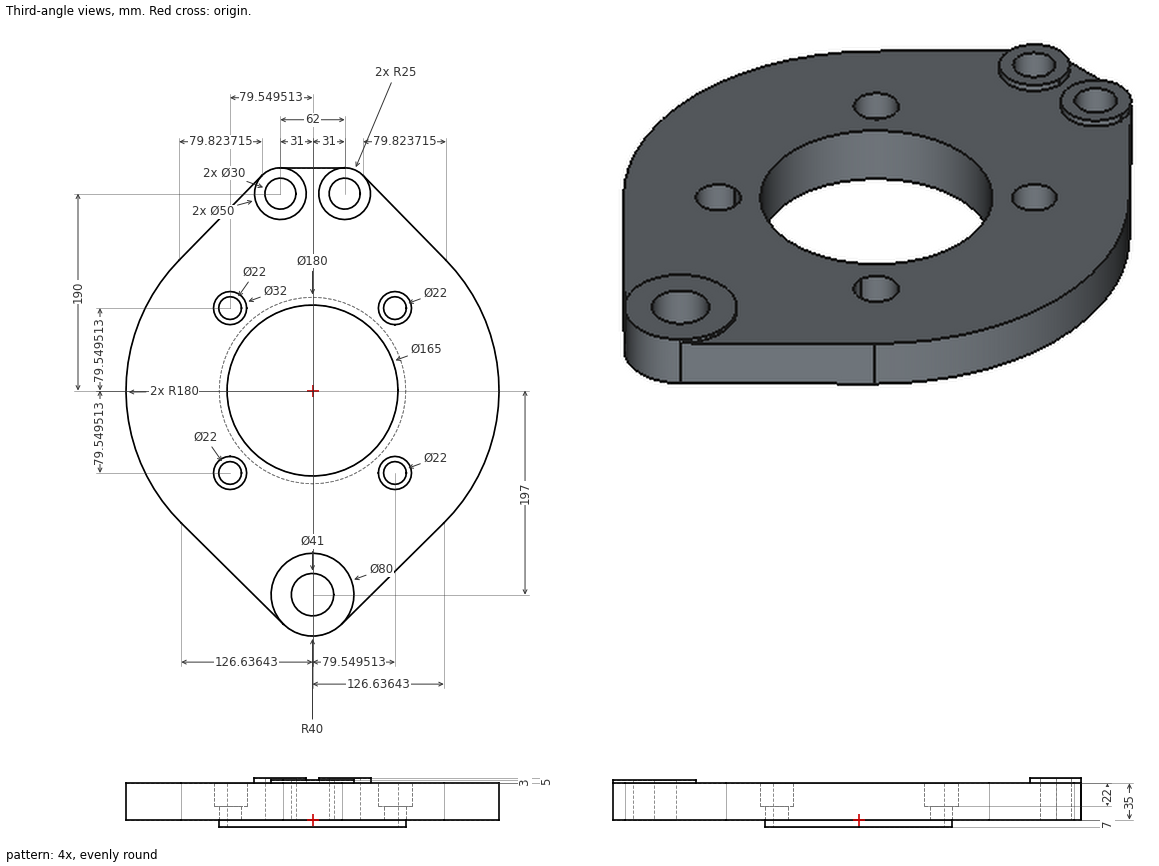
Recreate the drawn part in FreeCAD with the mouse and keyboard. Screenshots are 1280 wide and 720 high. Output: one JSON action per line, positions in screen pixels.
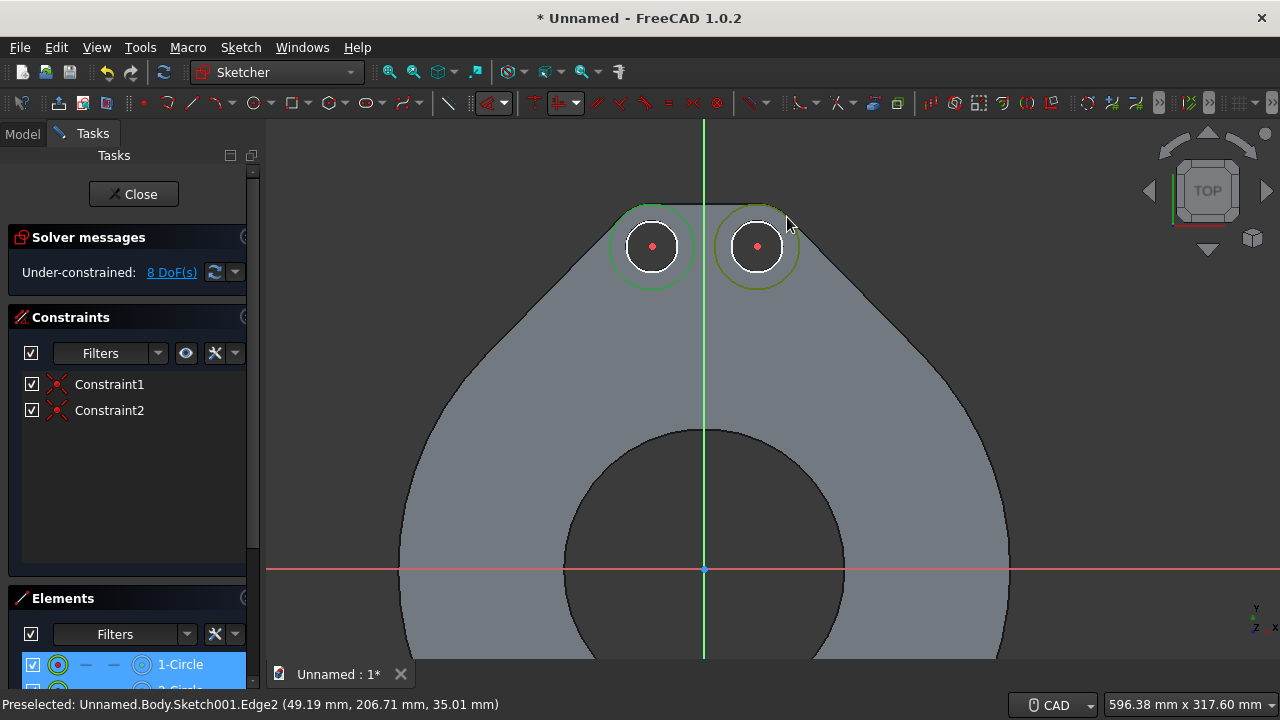
{"action": "left_click", "coordinate": [670, 104]}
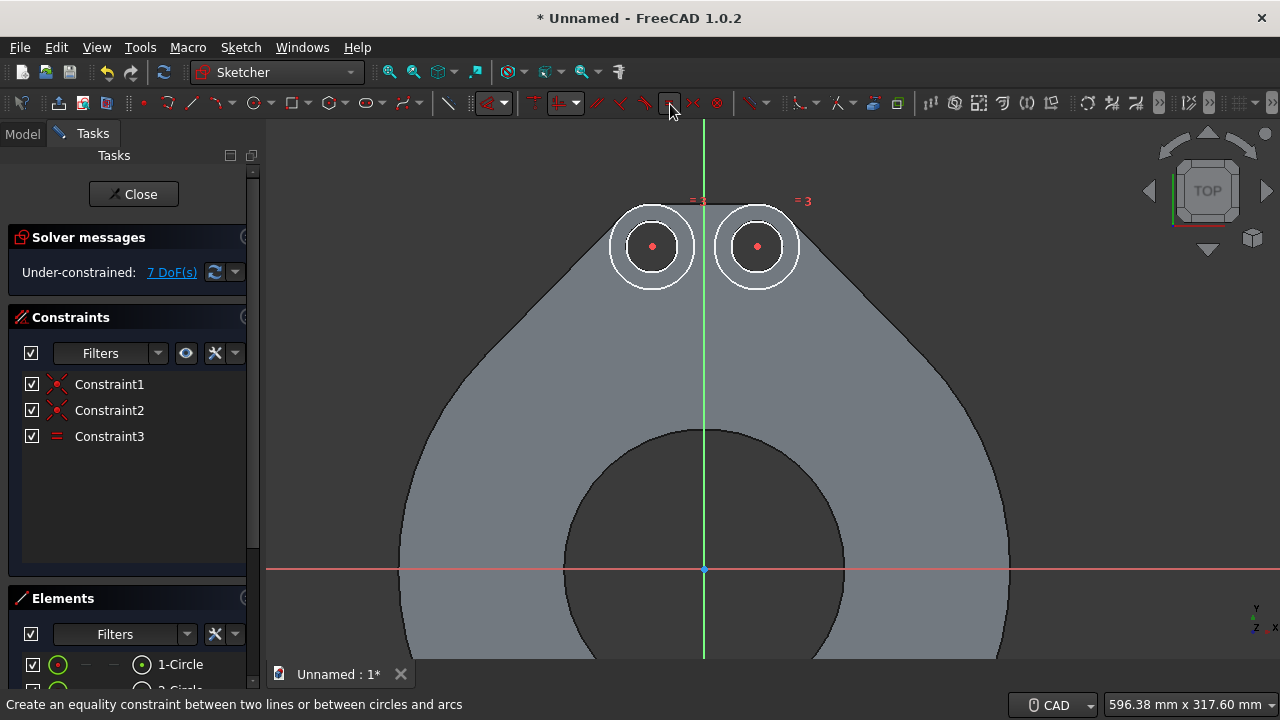
{"action": "left_click", "coordinate": [670, 229]}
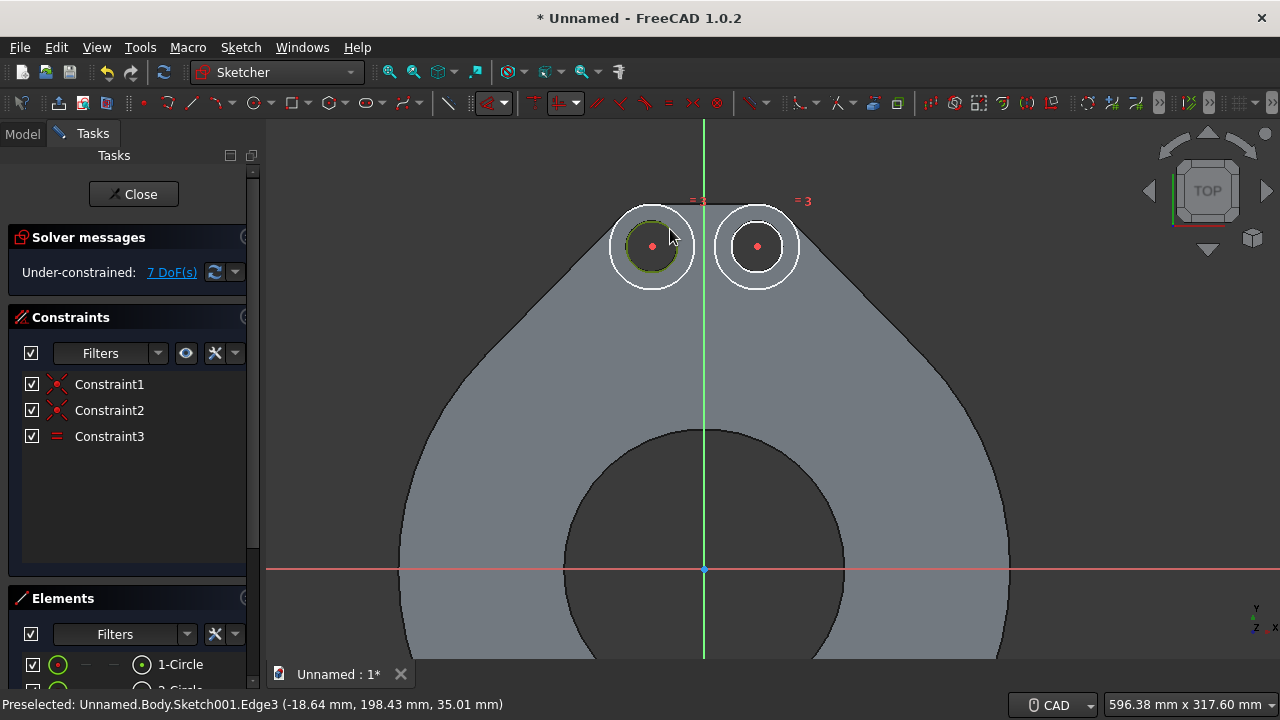
{"action": "left_click", "coordinate": [775, 229]}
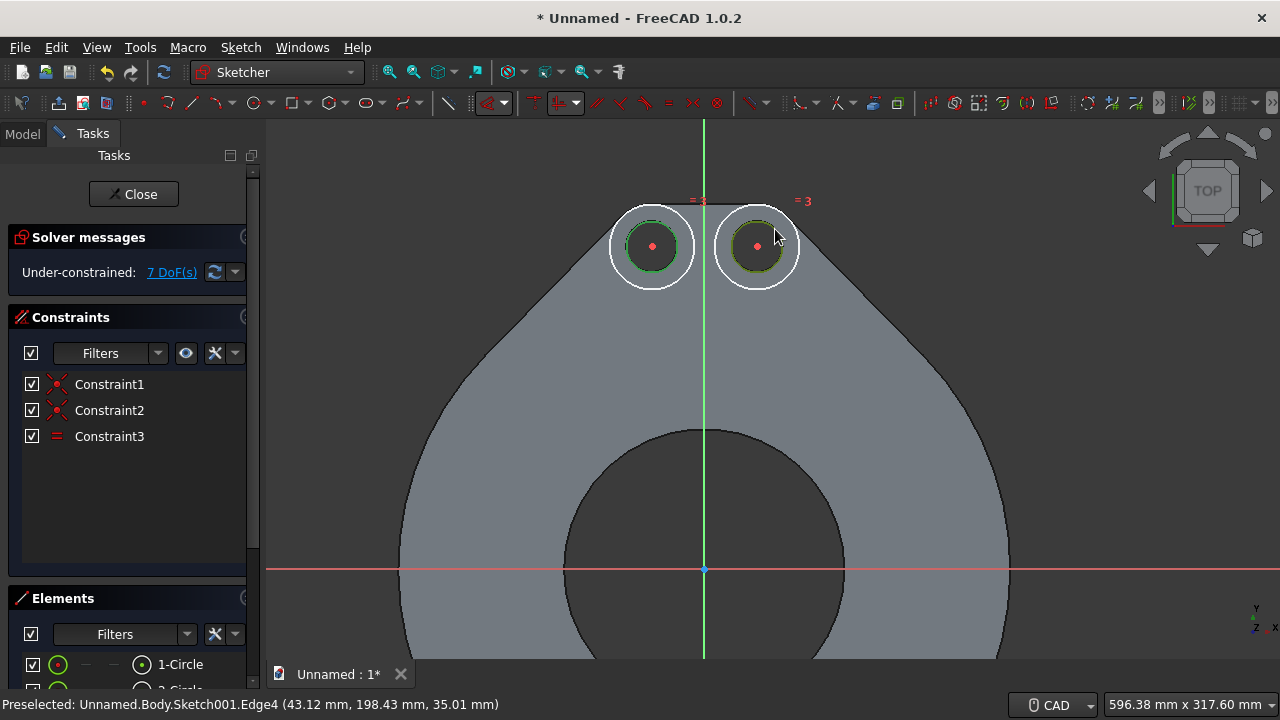
{"action": "key", "text": "e"}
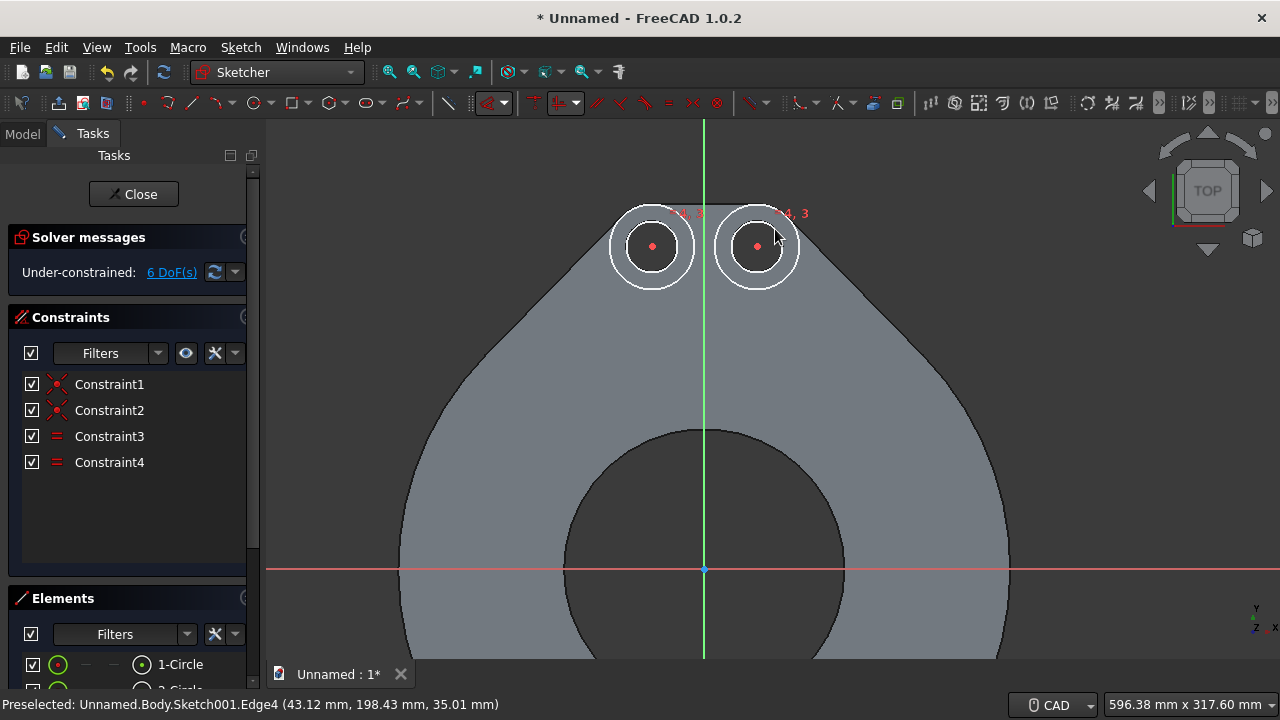
{"action": "left_click", "coordinate": [652, 247]}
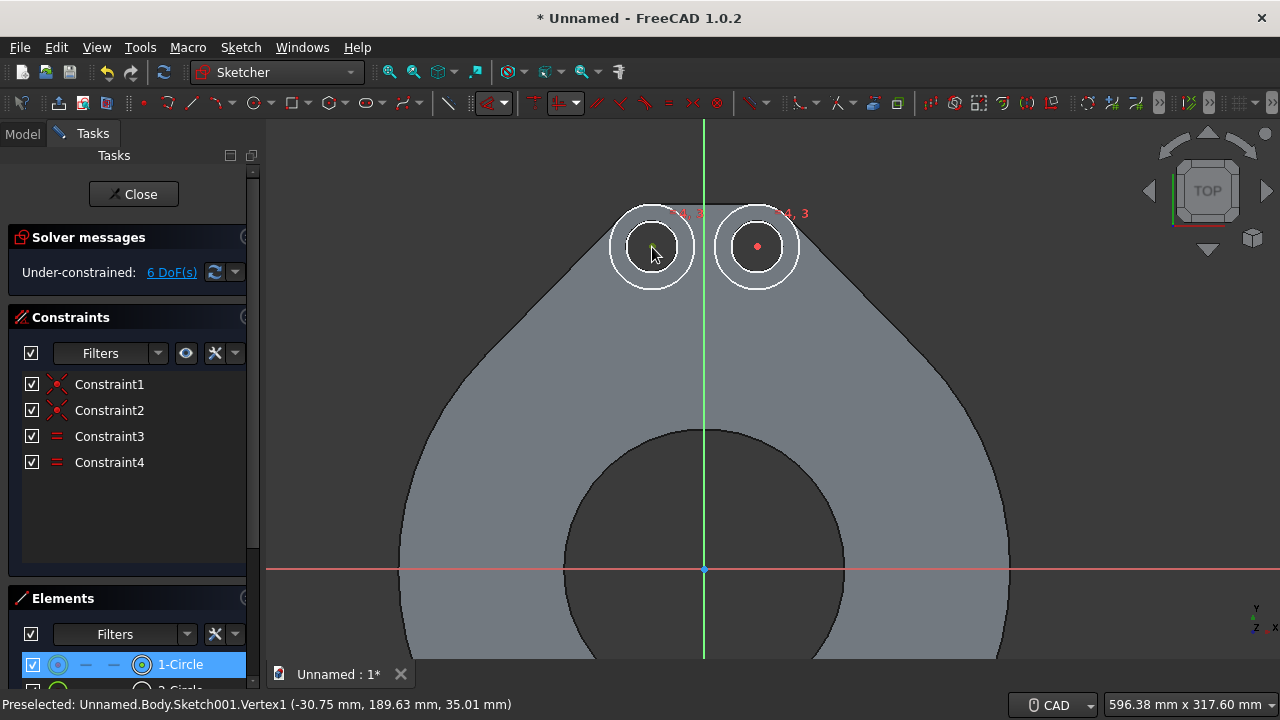
{"action": "left_click", "coordinate": [757, 247]}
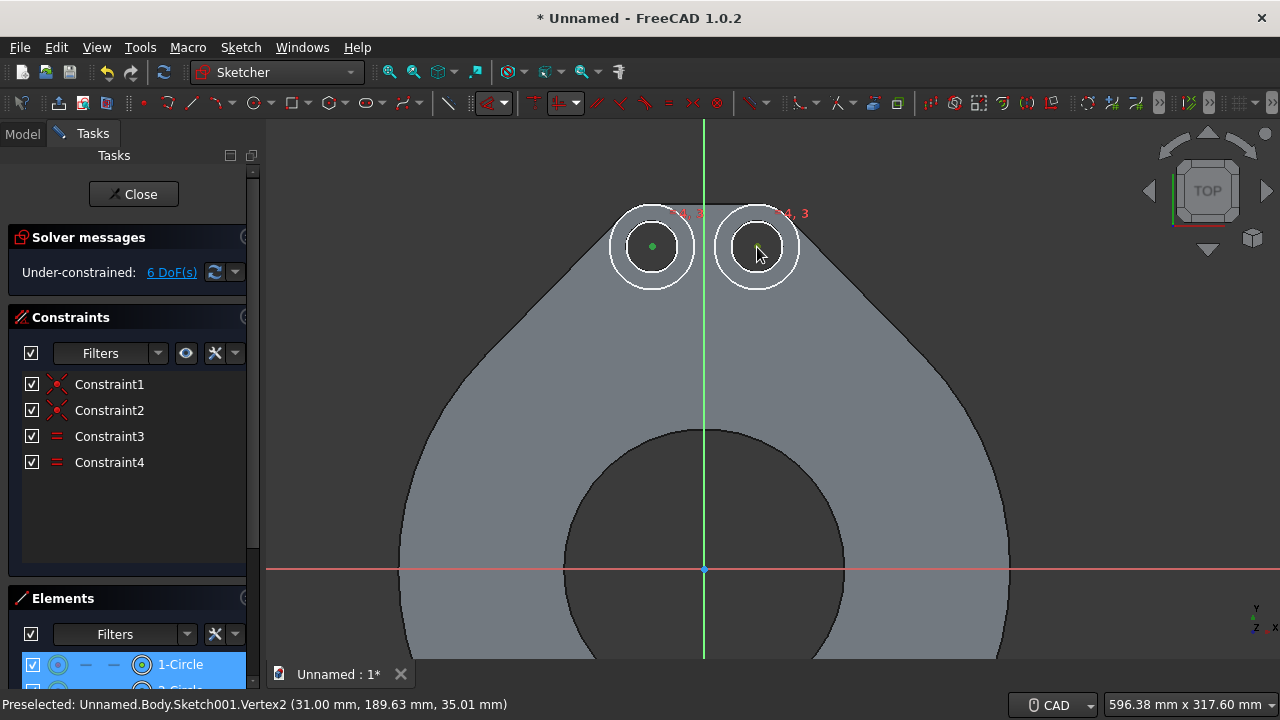
{"action": "key", "text": "h"}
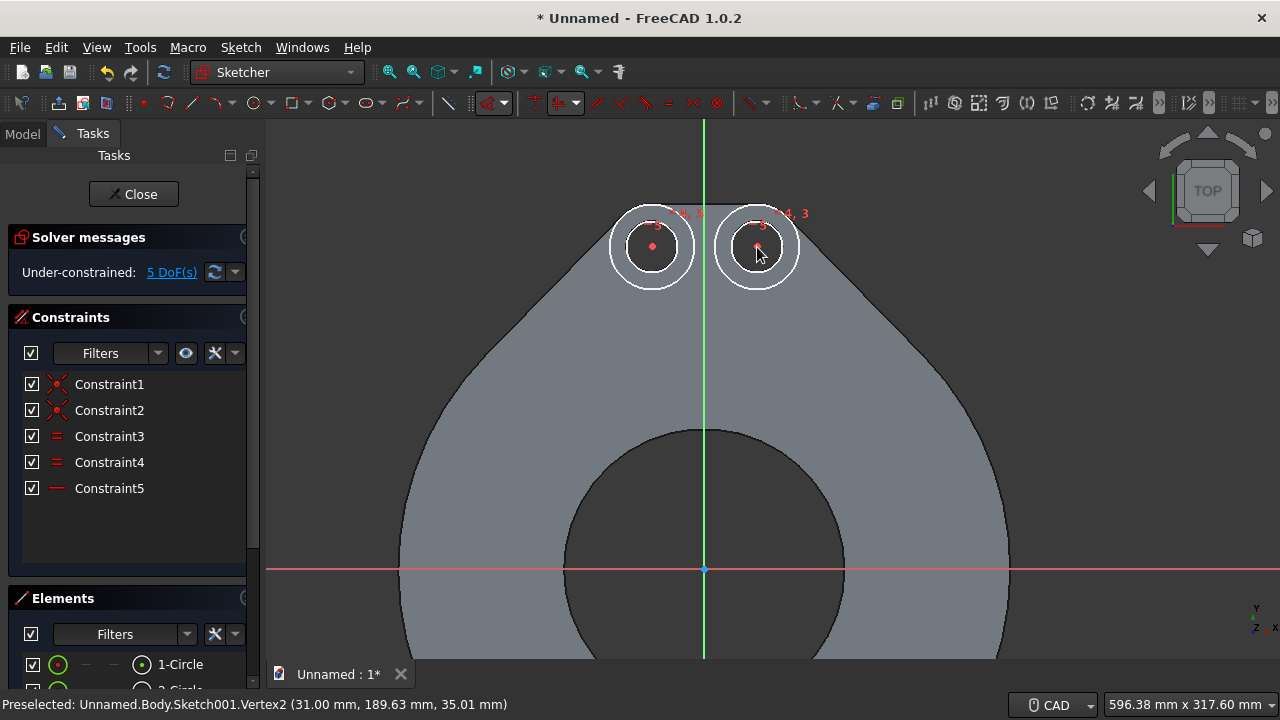
{"action": "left_click", "coordinate": [622, 217]}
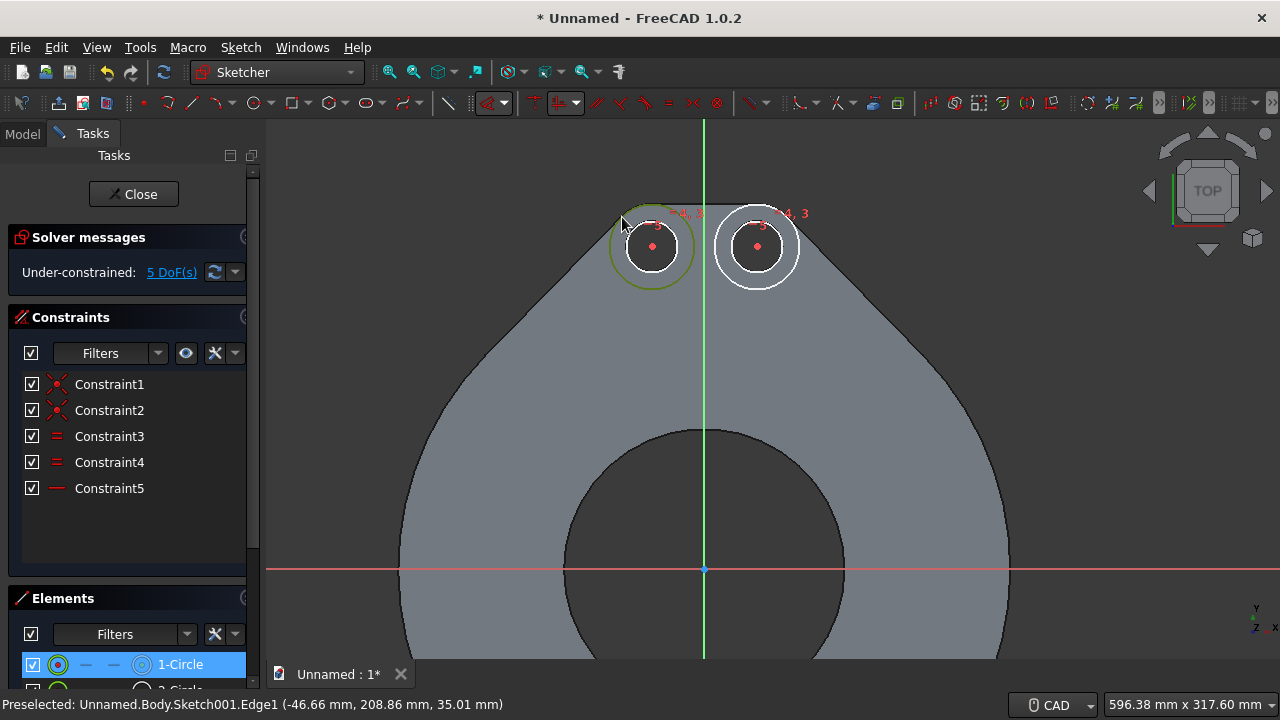
{"action": "key", "text": "k o"}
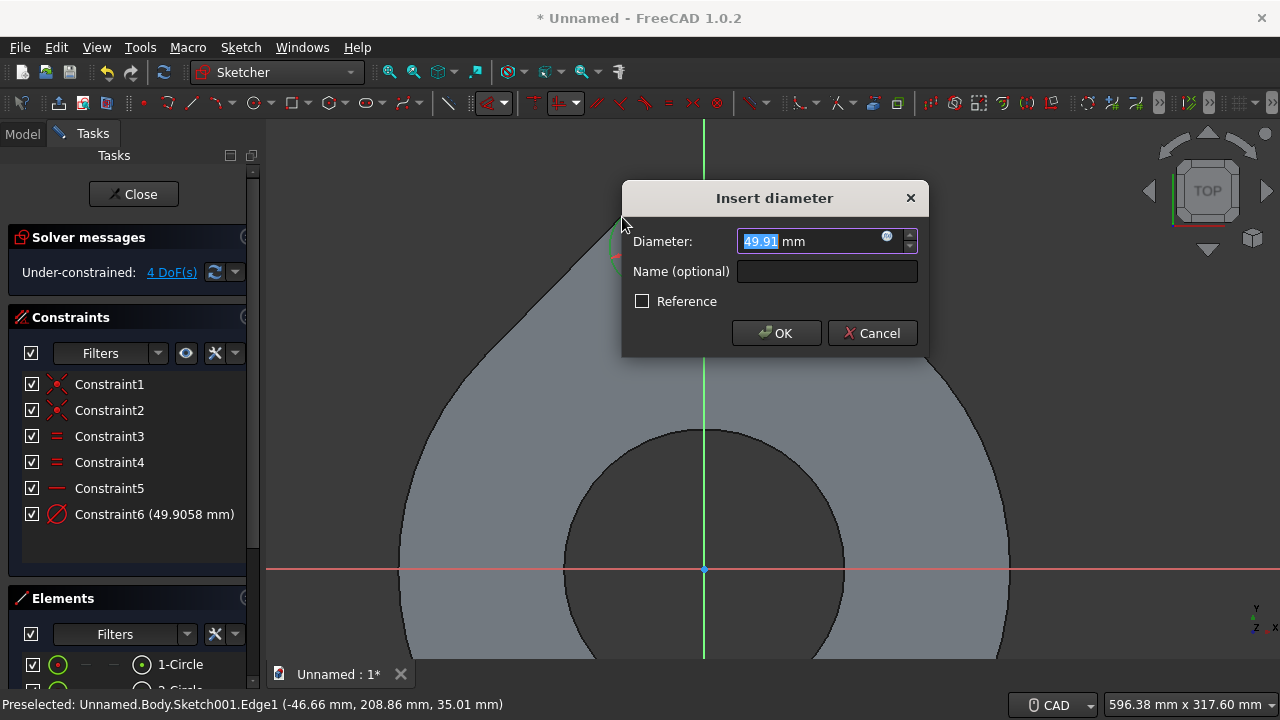
{"action": "type", "text": "50"}
{"action": "key", "text": "Return"}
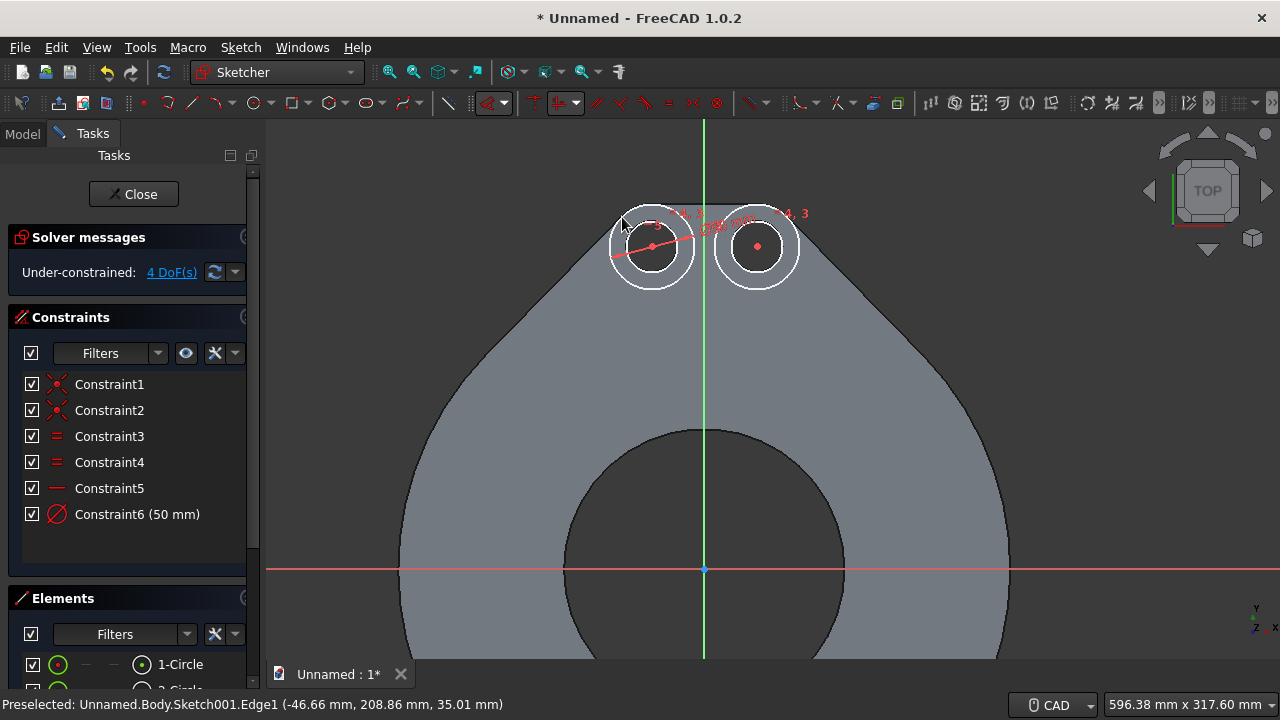
{"action": "left_click", "coordinate": [670, 229]}